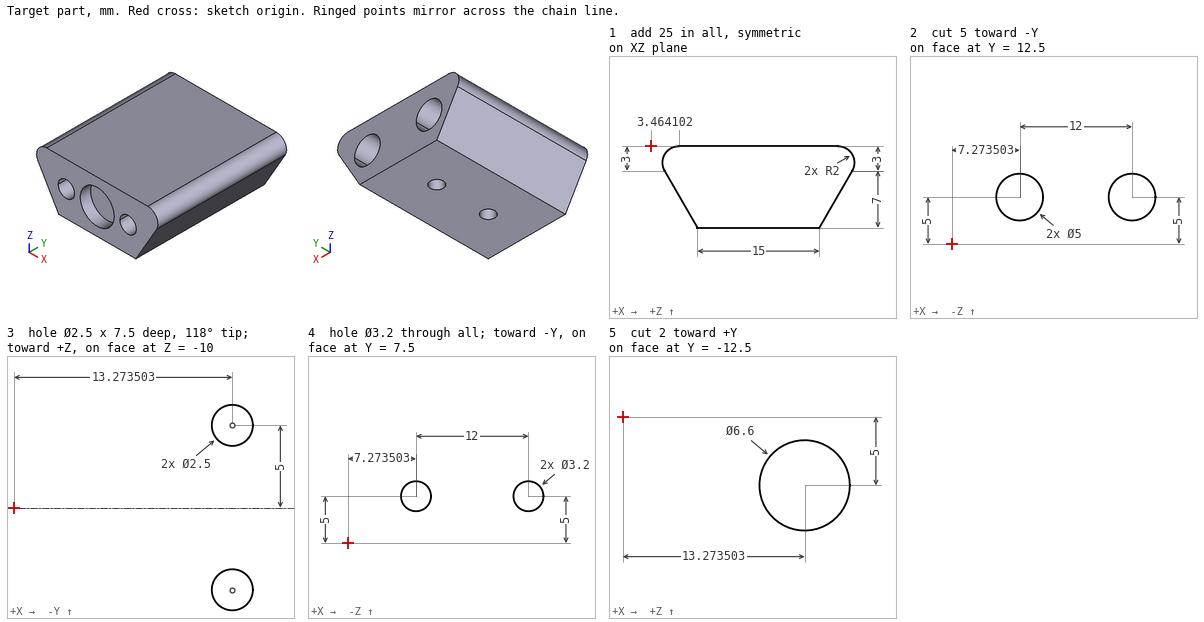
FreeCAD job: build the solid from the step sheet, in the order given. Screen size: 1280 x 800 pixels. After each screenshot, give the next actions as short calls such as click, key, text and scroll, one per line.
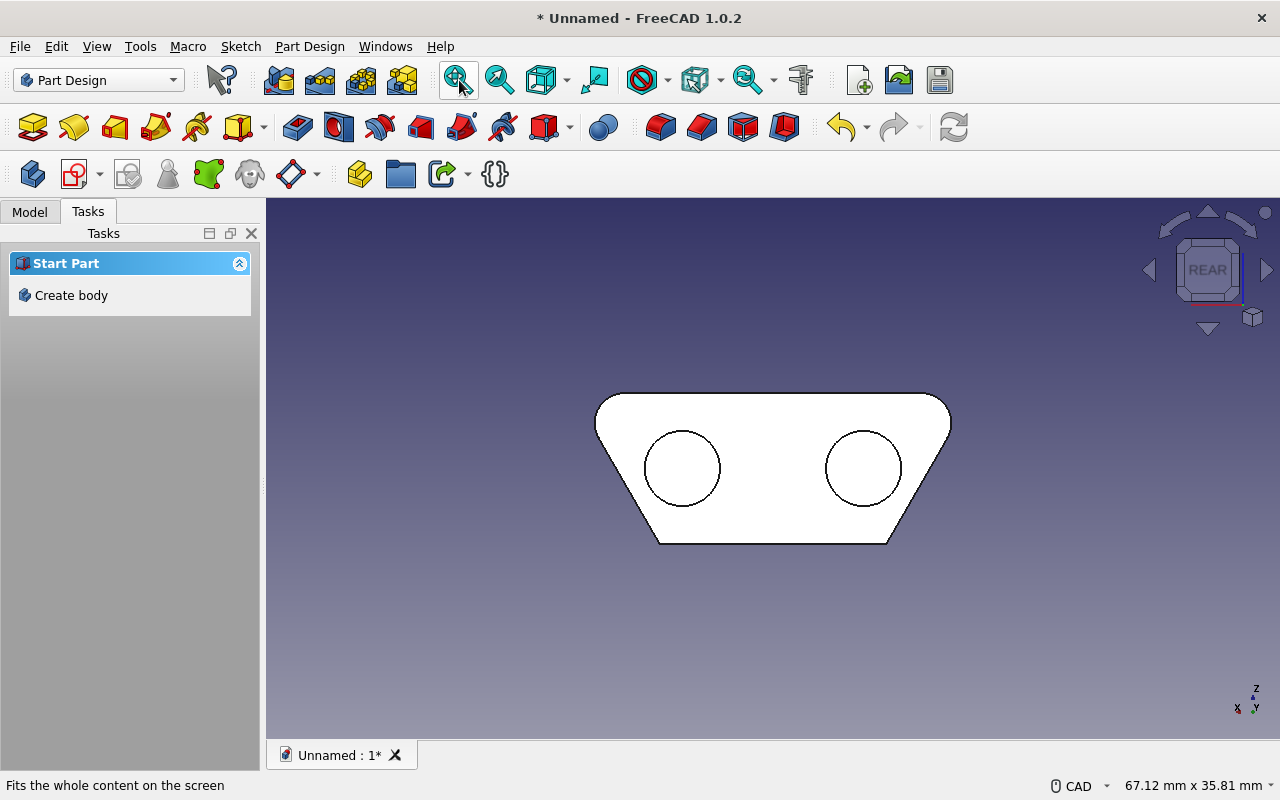
key(5)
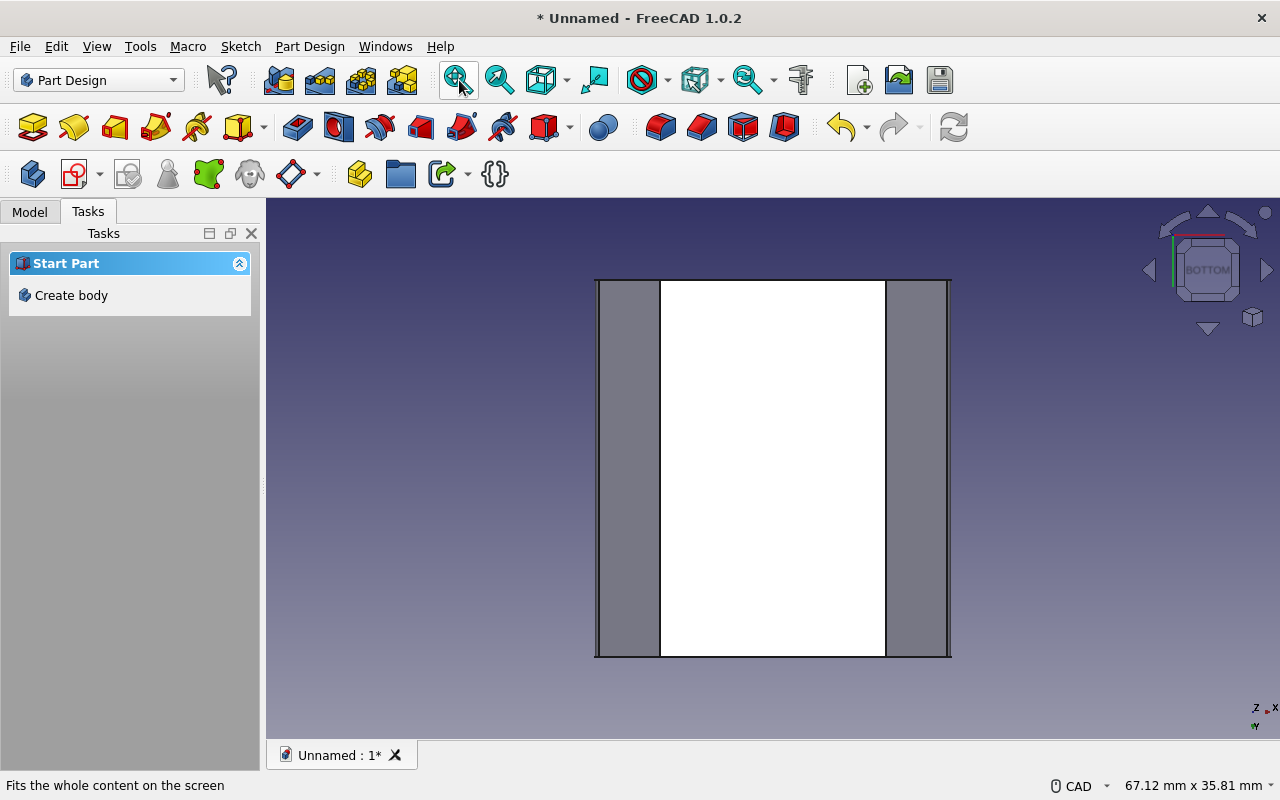
click(773, 521)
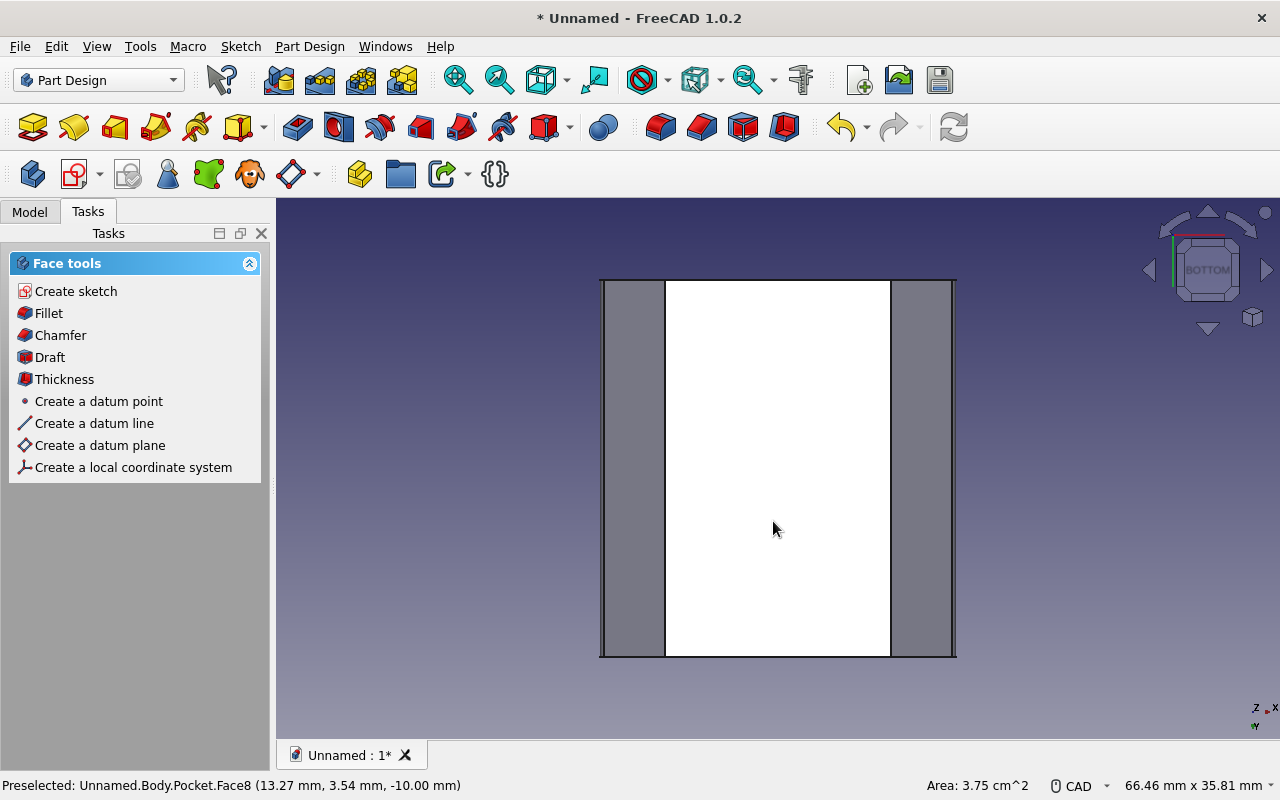
click(74, 174)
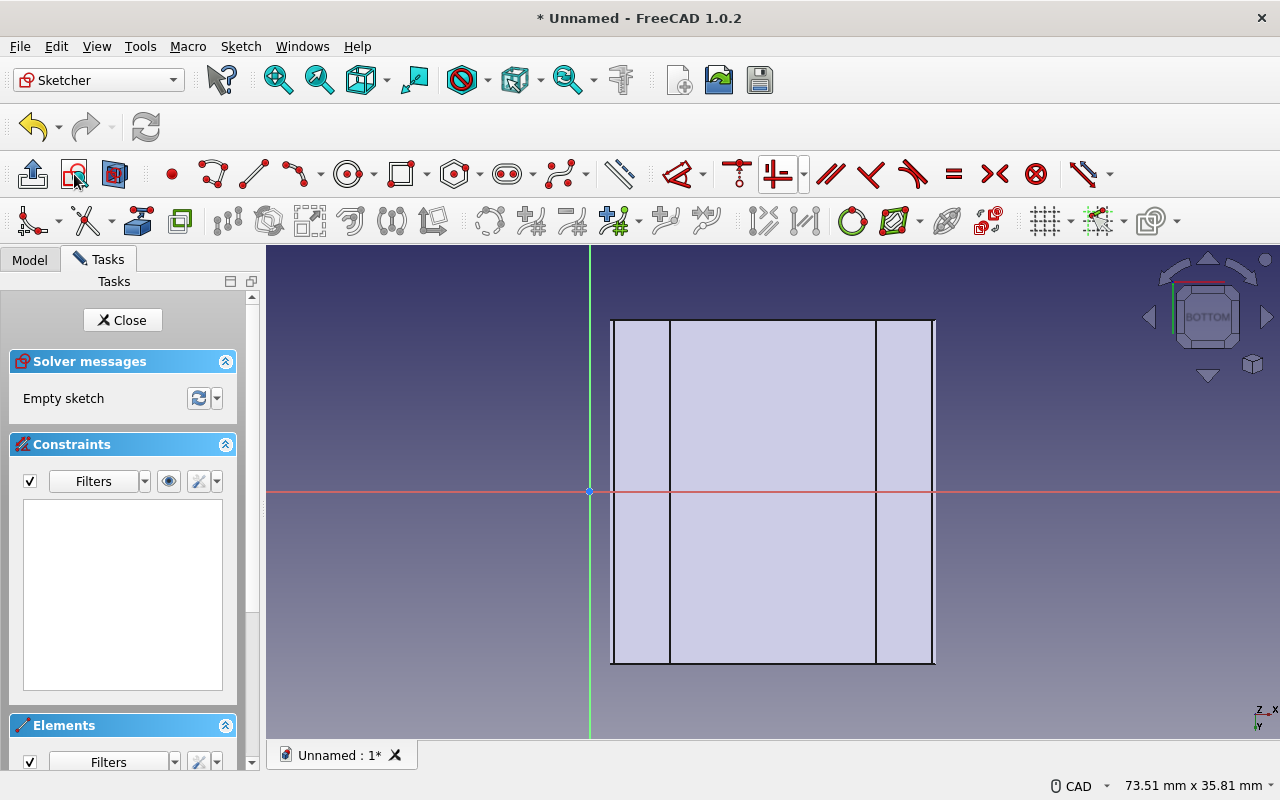
scroll(673, 492, up, 3)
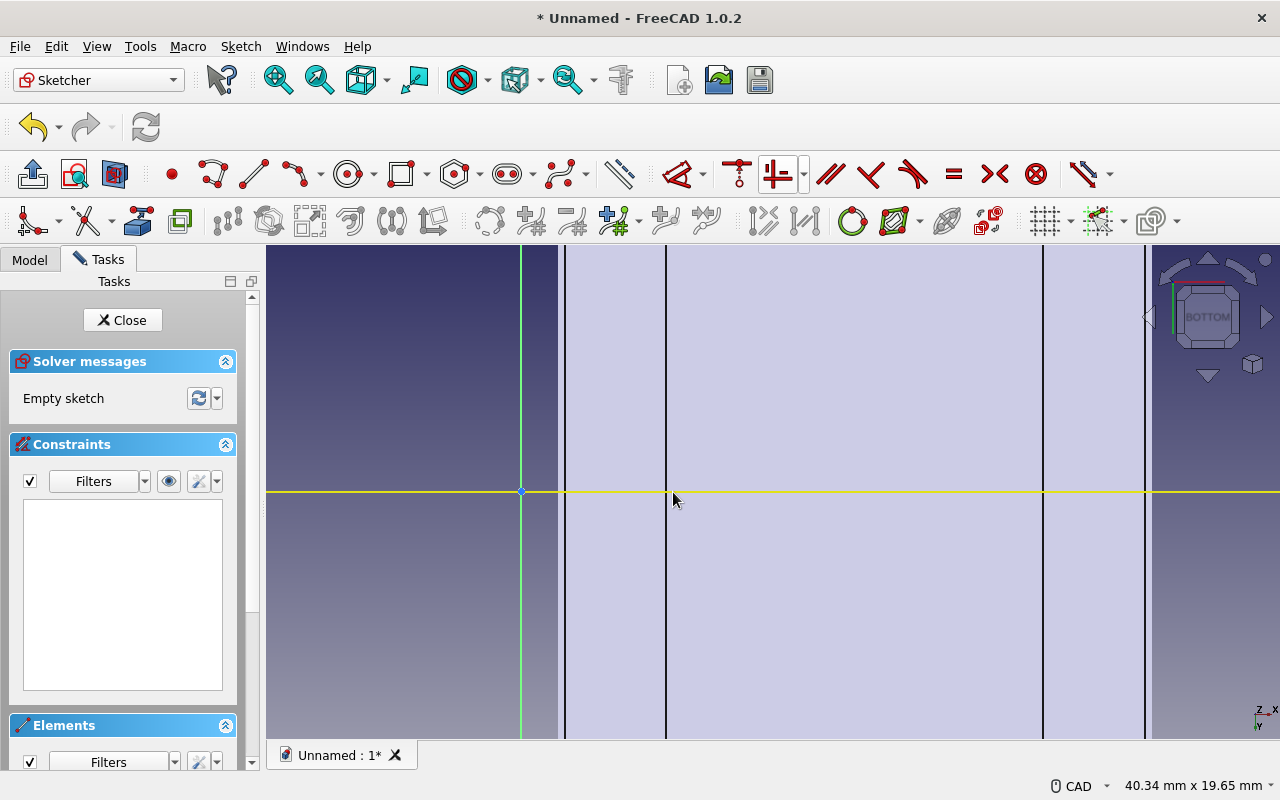
click(348, 174)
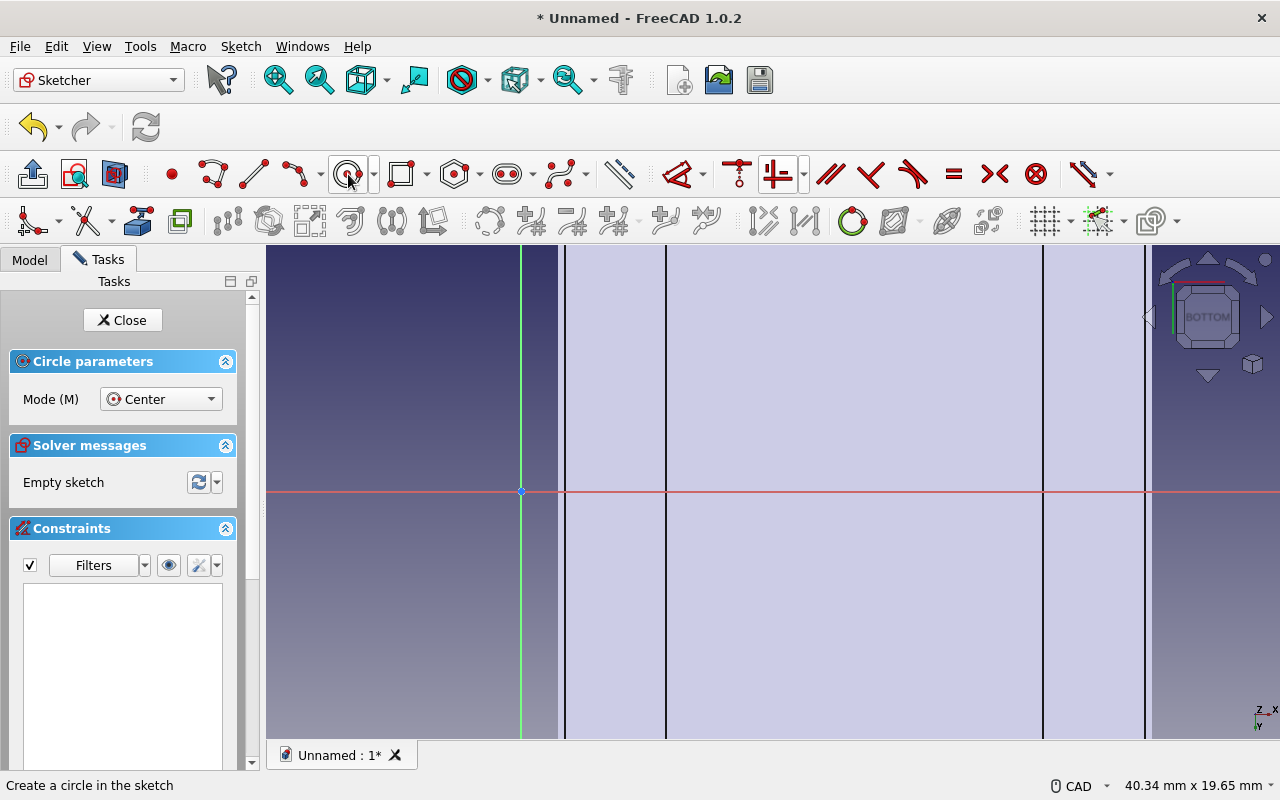
click(855, 366)
click(877, 344)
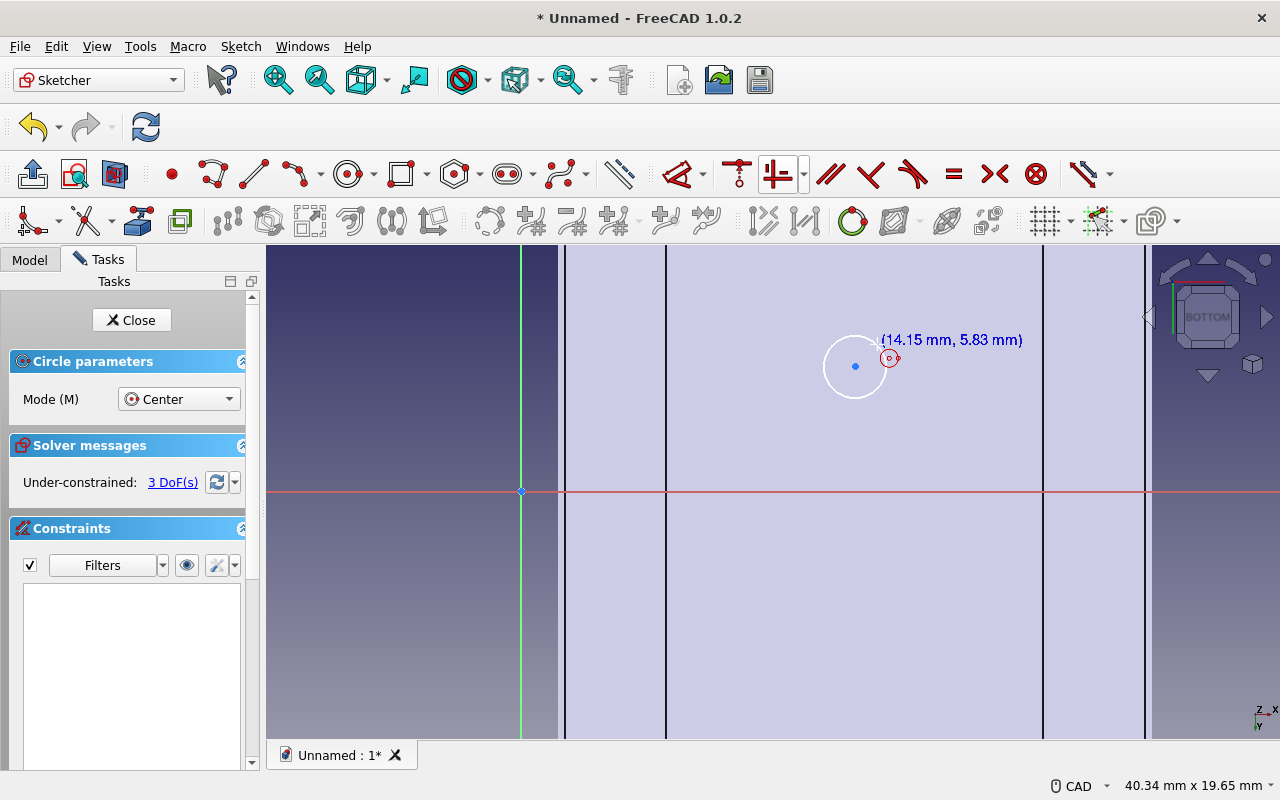
click(855, 617)
click(877, 595)
key(Escape)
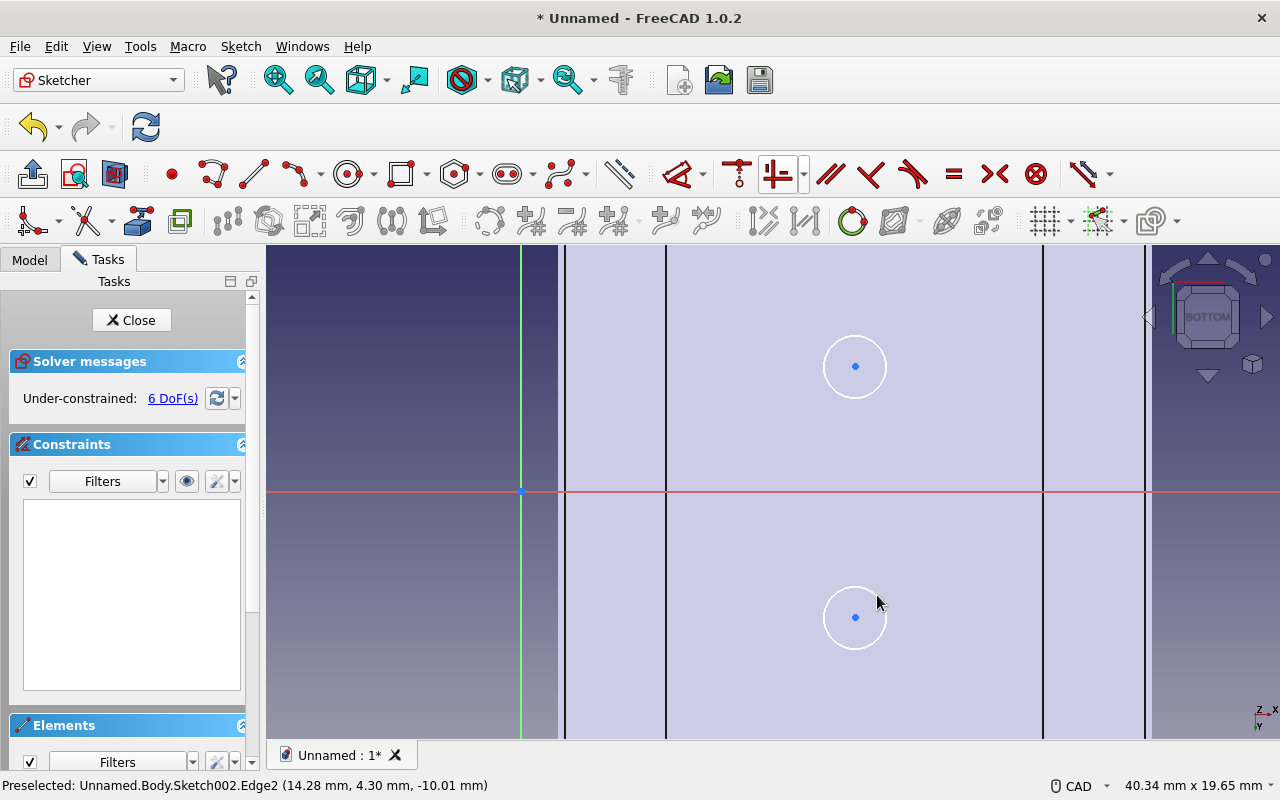
click(877, 345)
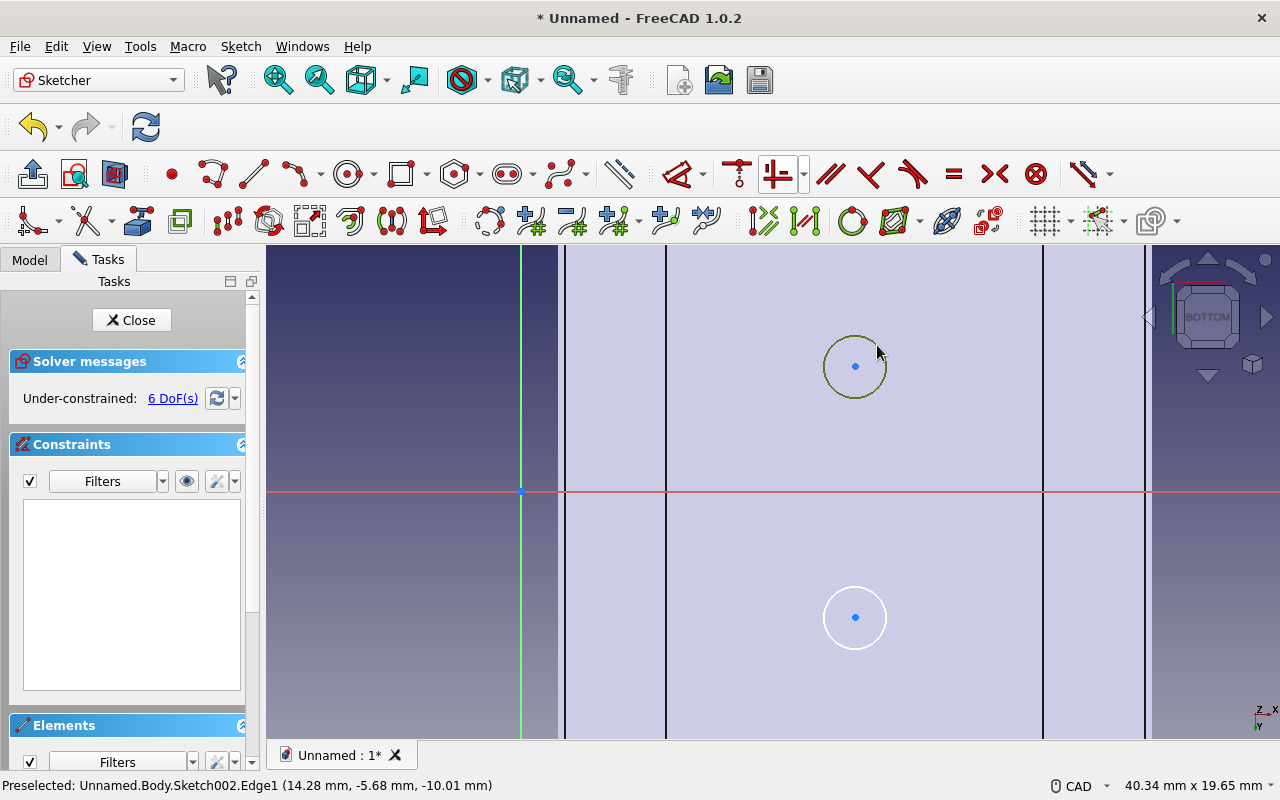
click(877, 596)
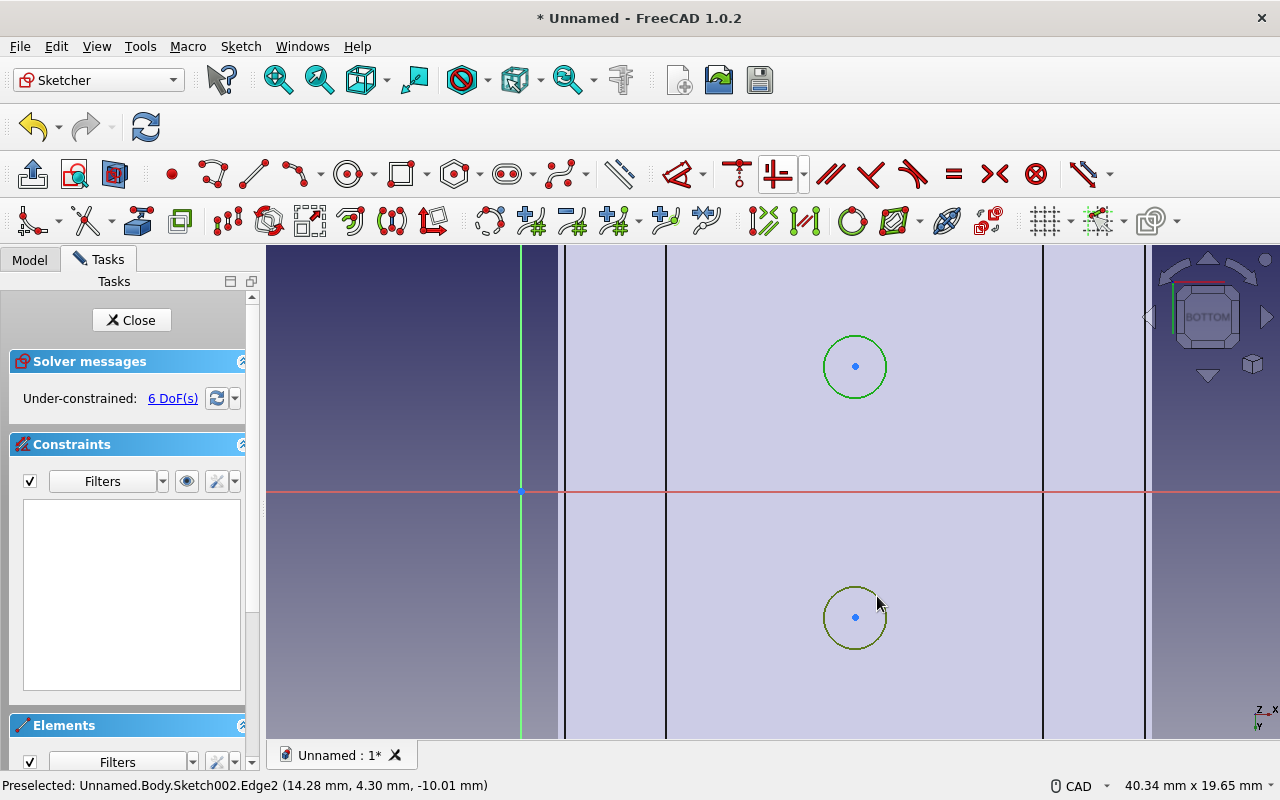
click(954, 174)